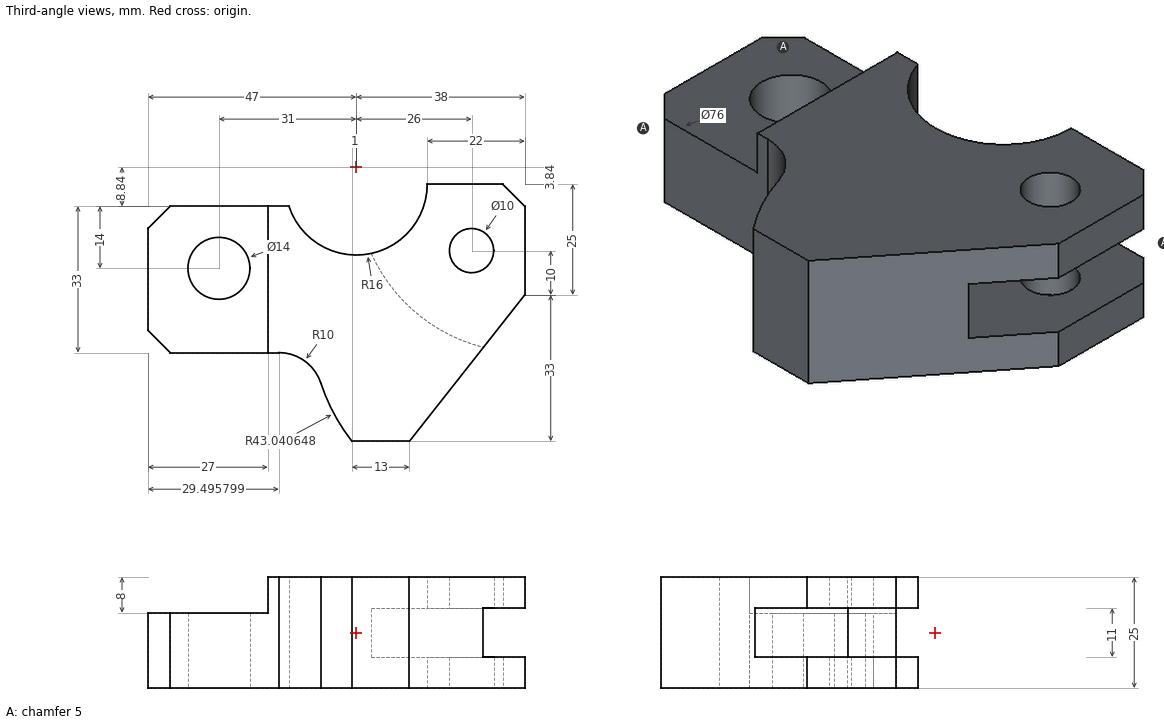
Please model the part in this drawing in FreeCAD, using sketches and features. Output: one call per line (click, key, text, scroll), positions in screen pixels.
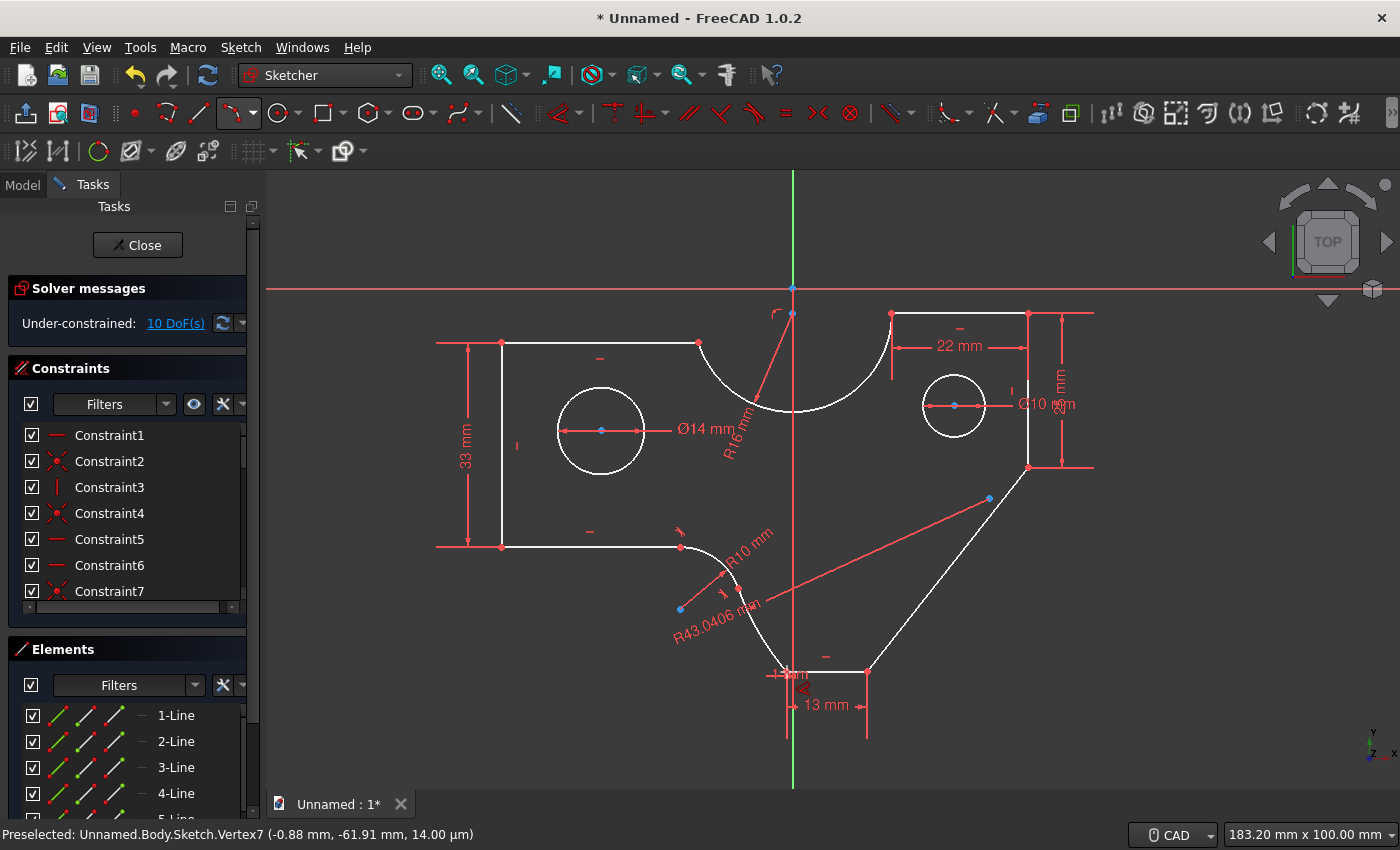
click(601, 431)
click(697, 255)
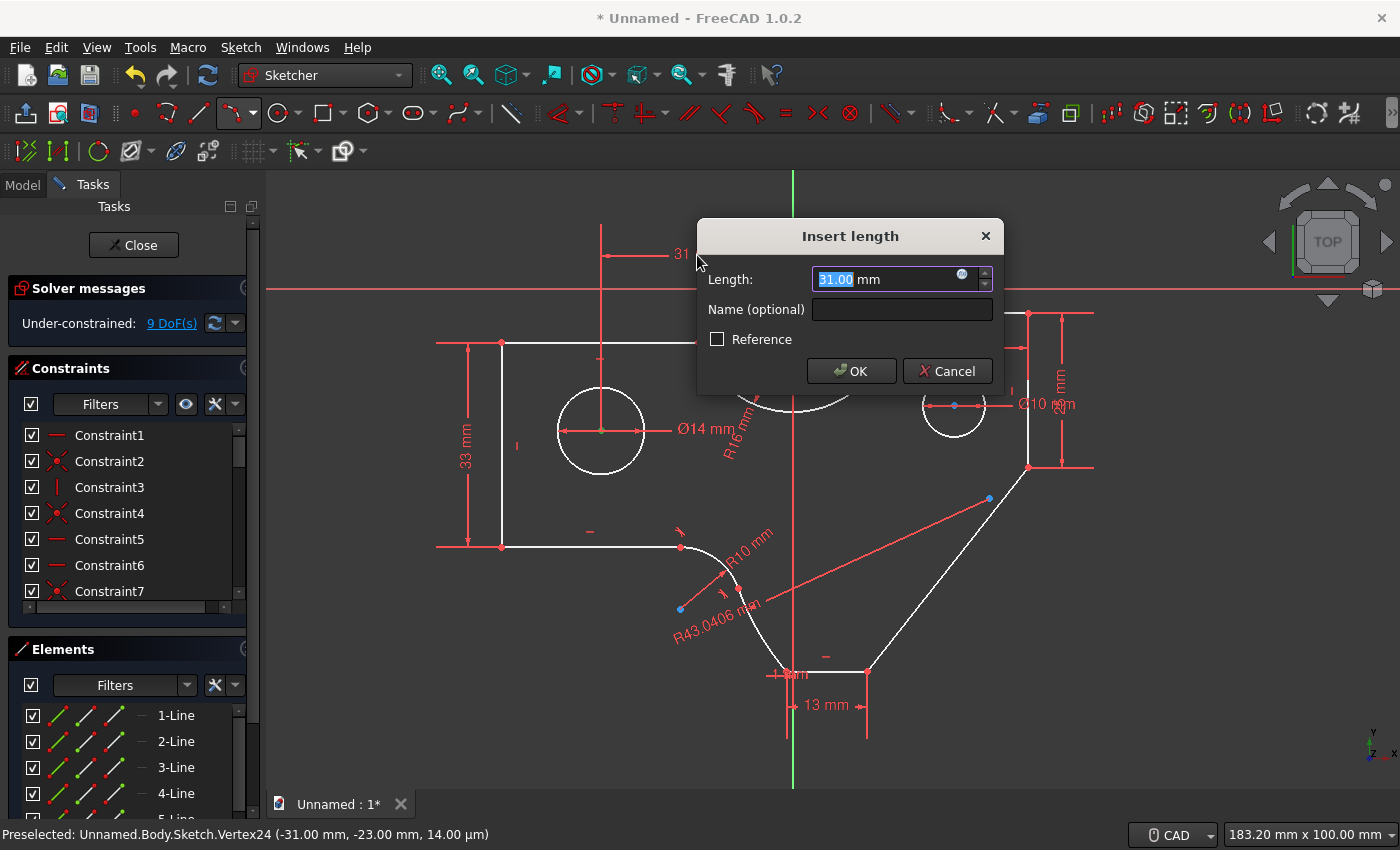
text(31)
key(Return)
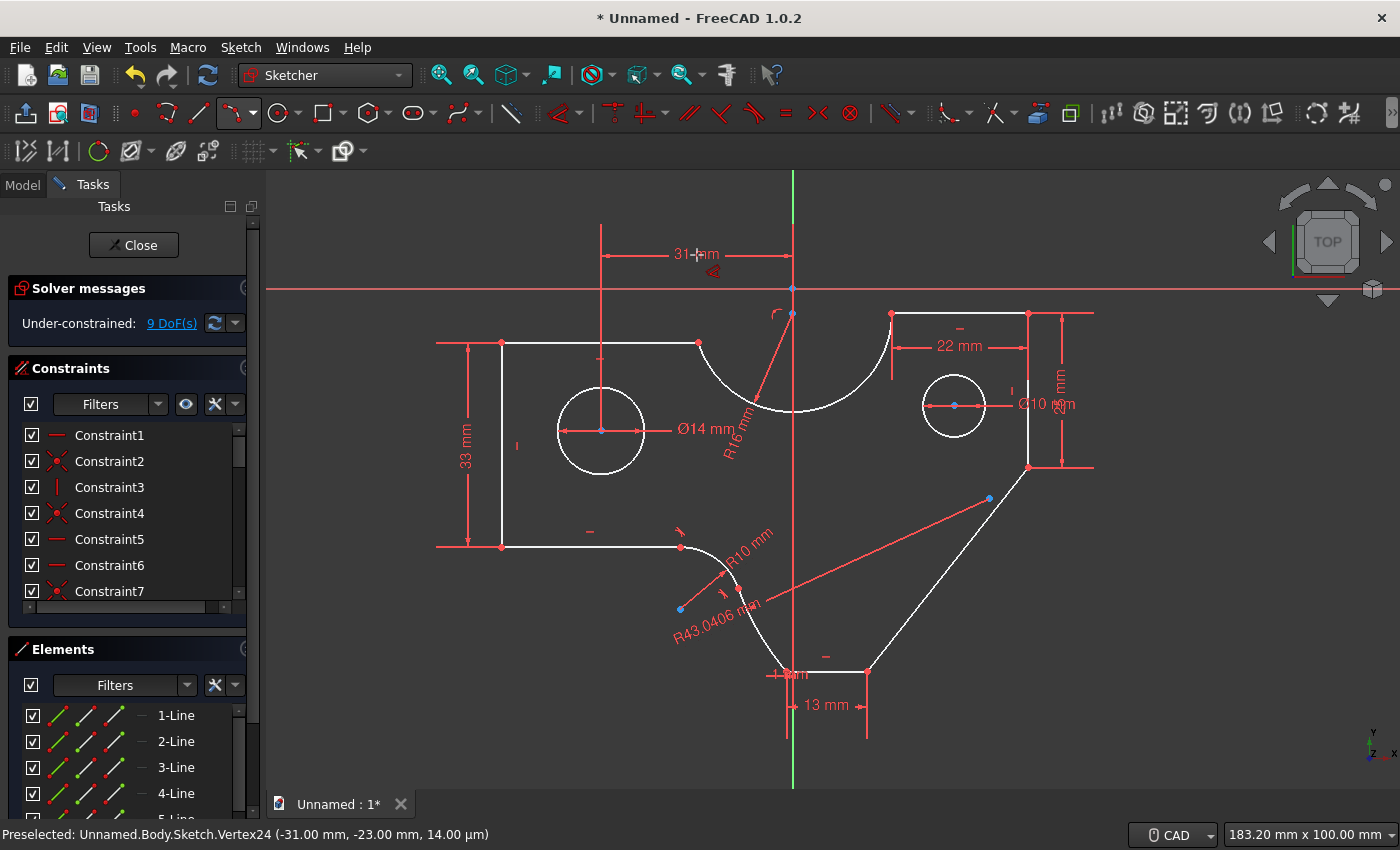
click(954, 406)
click(873, 255)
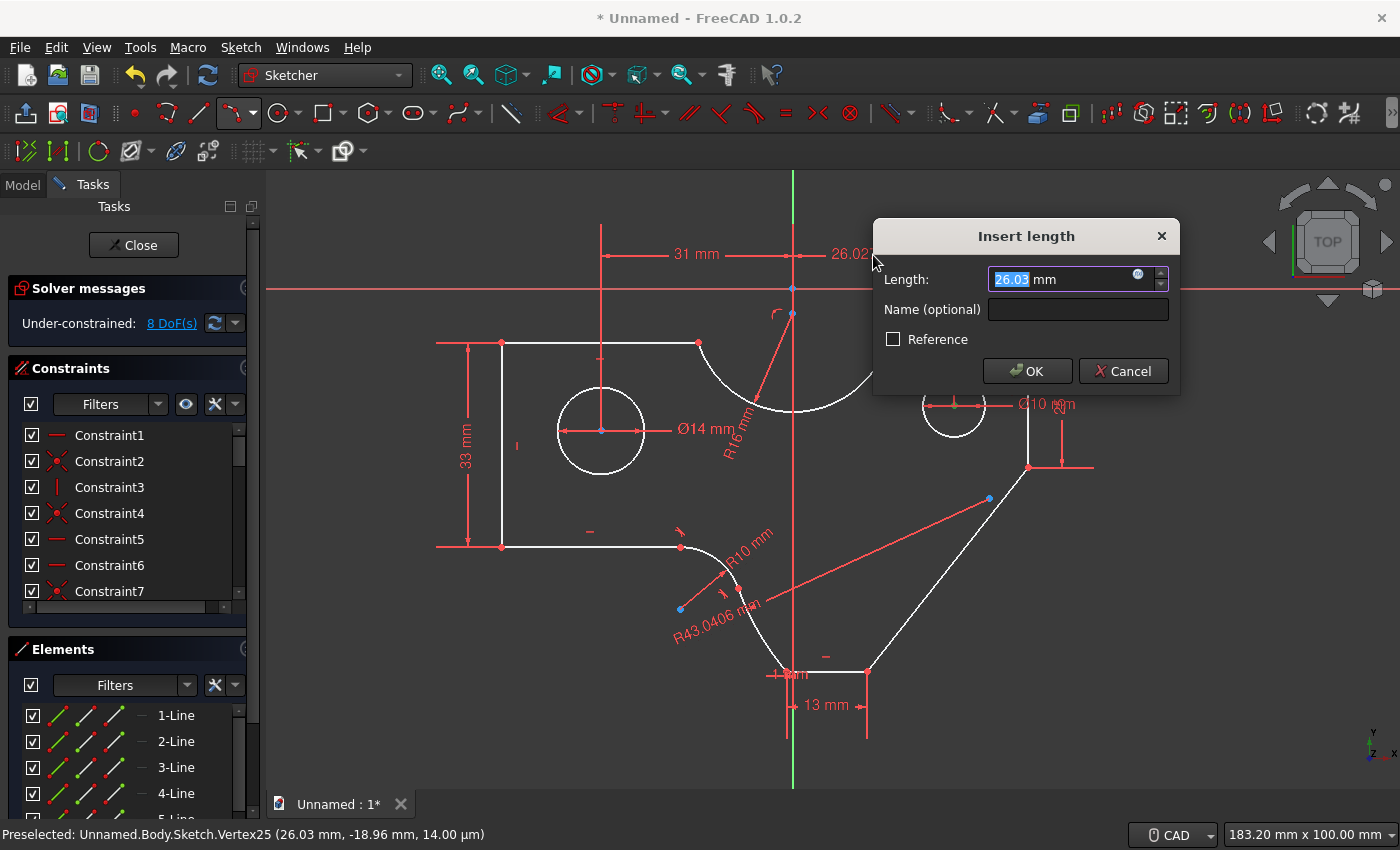
text(26)
key(Return)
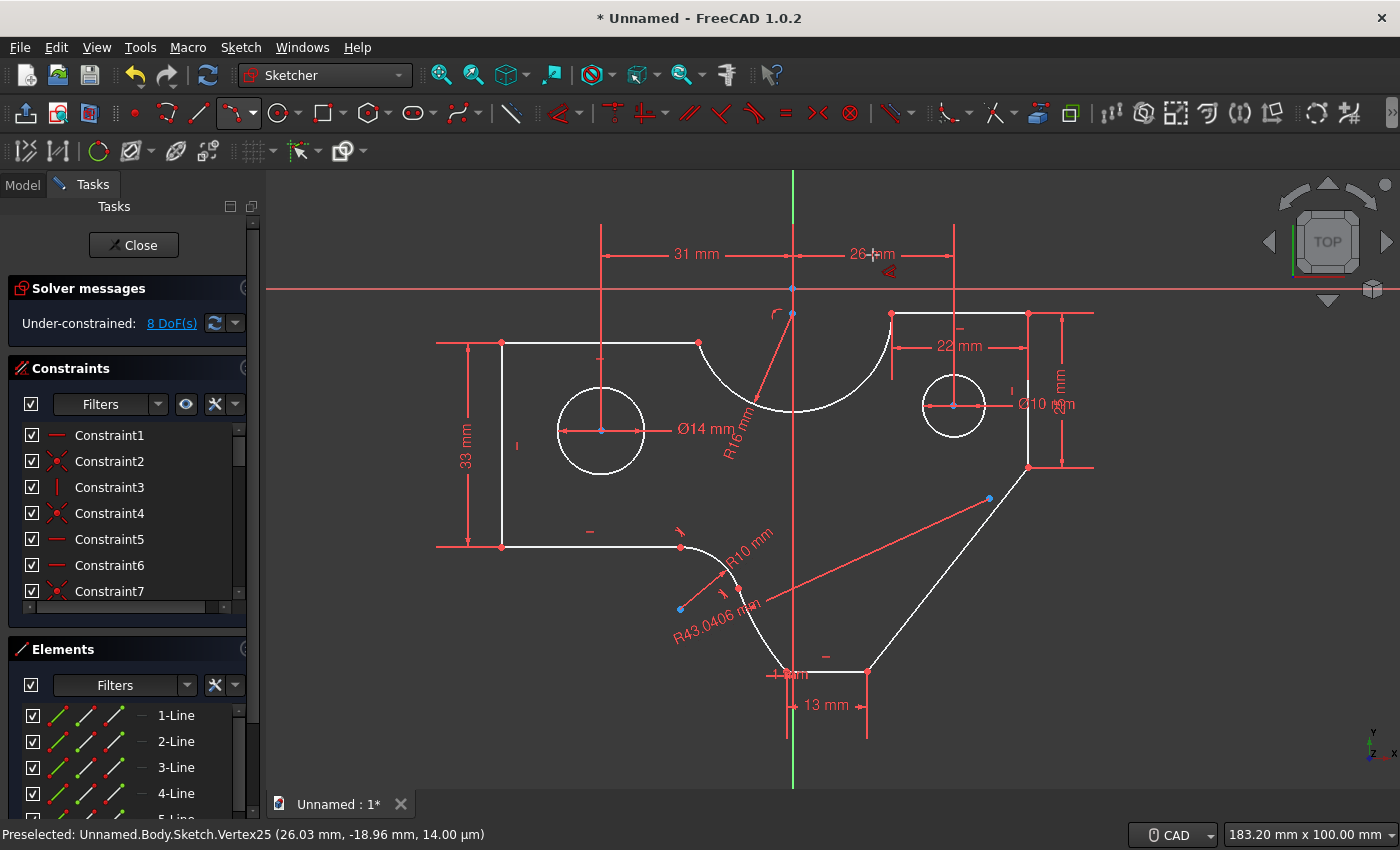
click(502, 343)
click(580, 255)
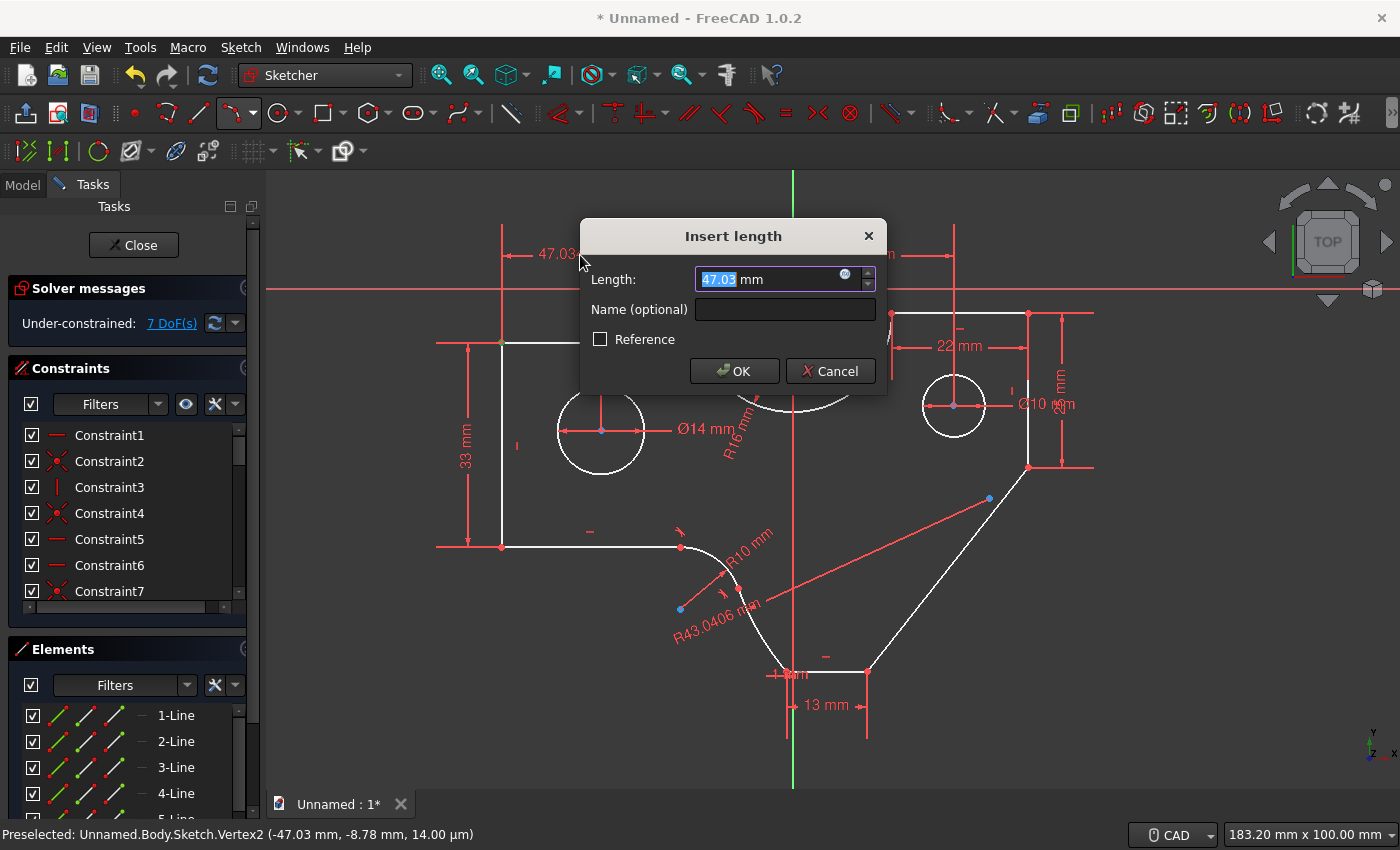
text(47)
key(Return)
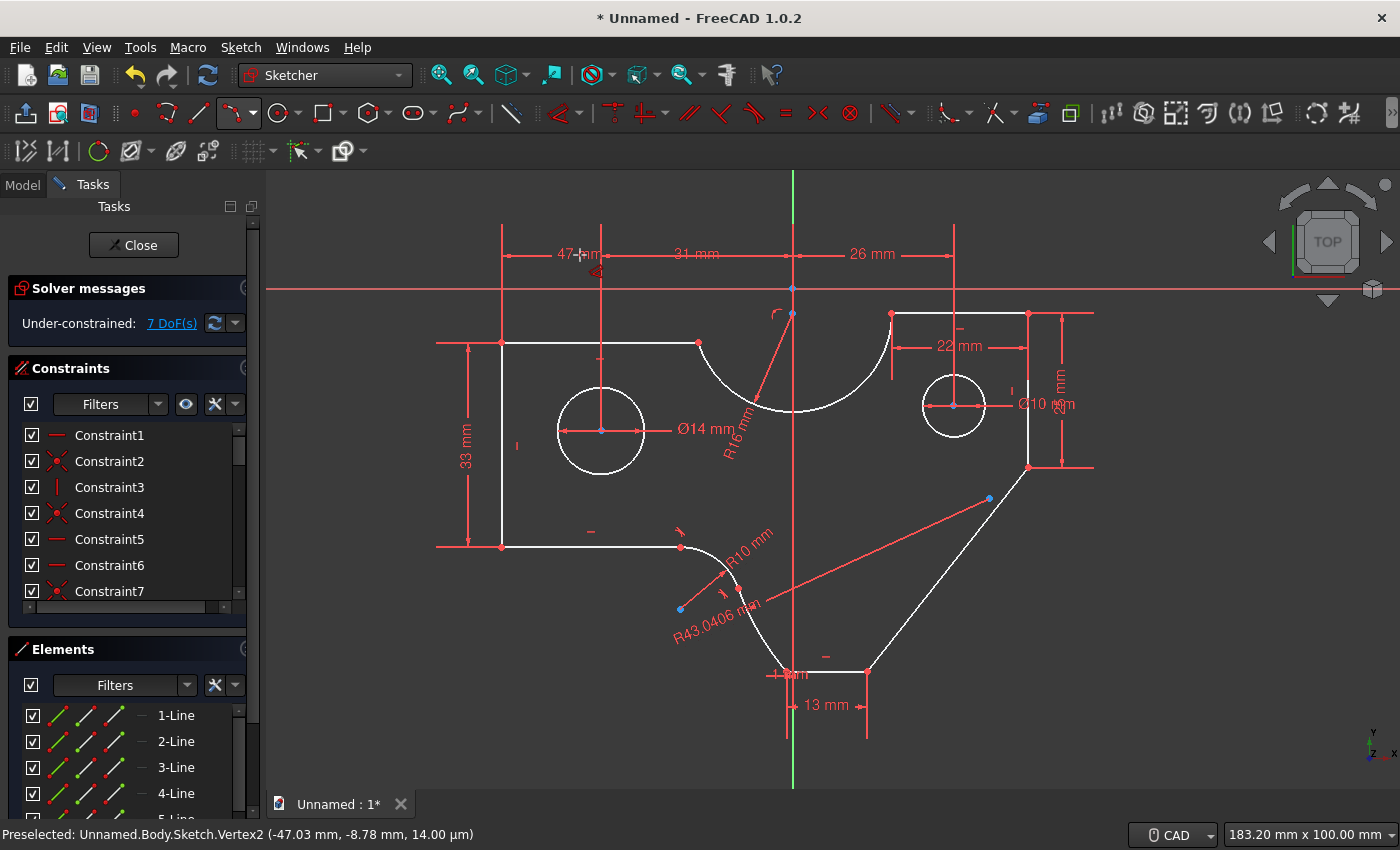
click(915, 611)
click(1062, 570)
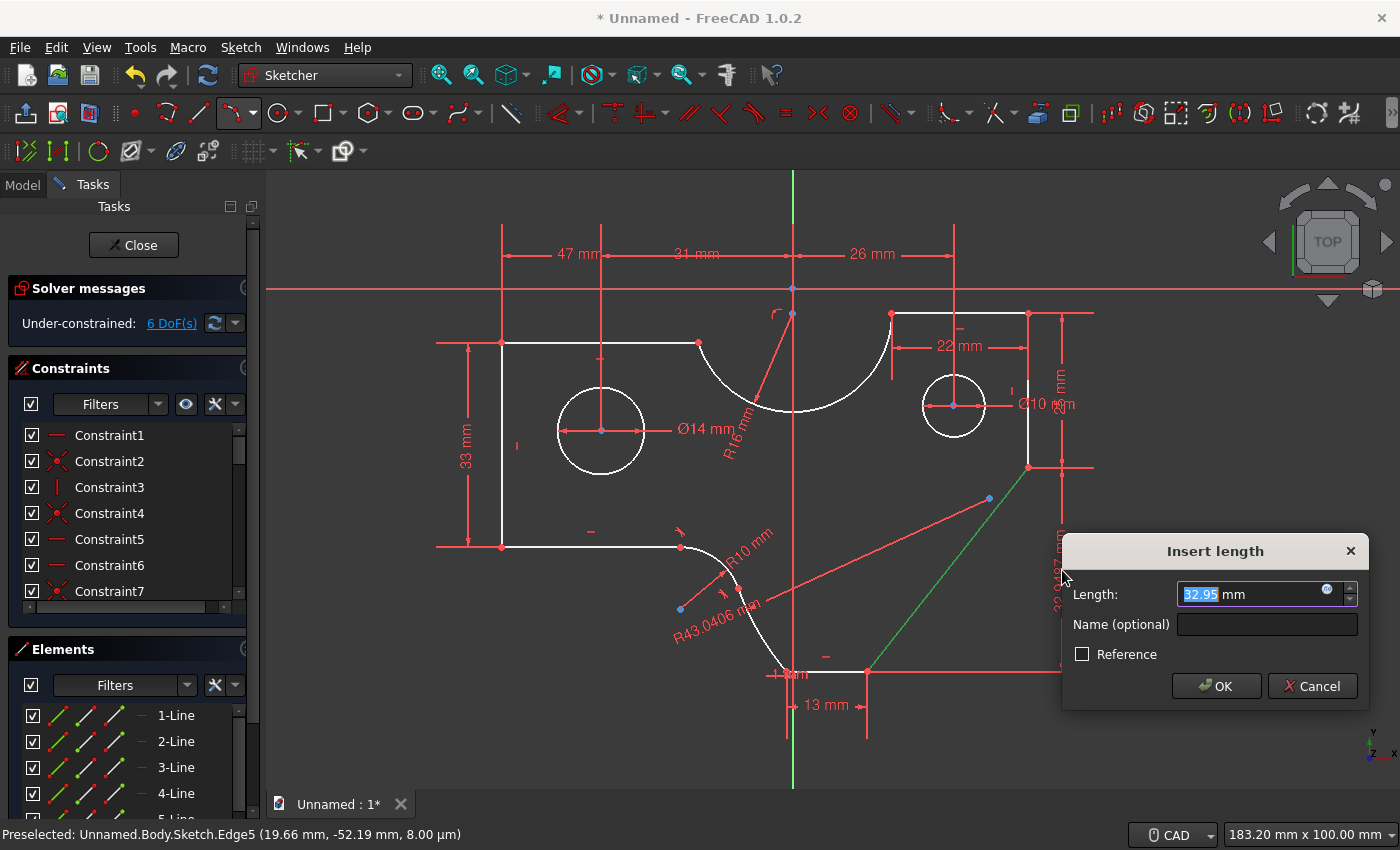
text(33)
key(Return)